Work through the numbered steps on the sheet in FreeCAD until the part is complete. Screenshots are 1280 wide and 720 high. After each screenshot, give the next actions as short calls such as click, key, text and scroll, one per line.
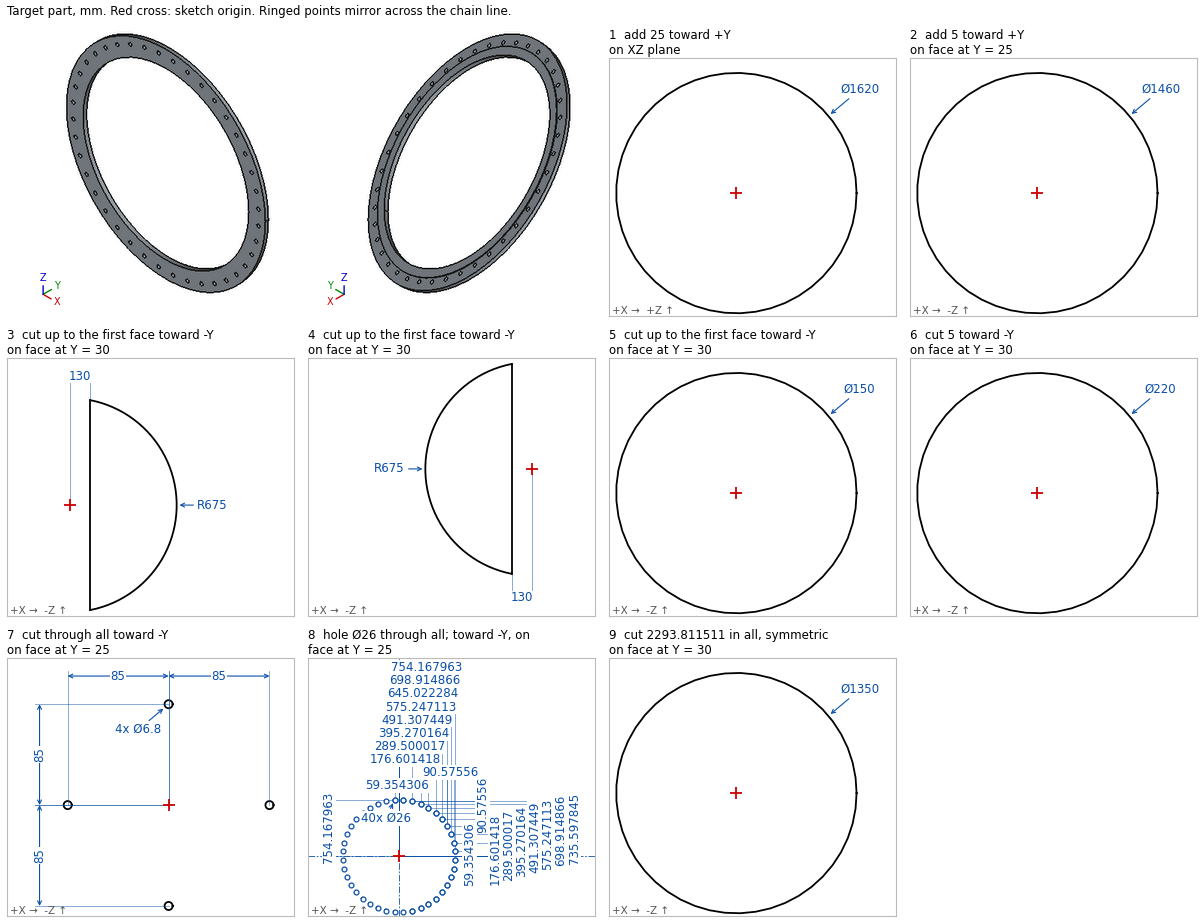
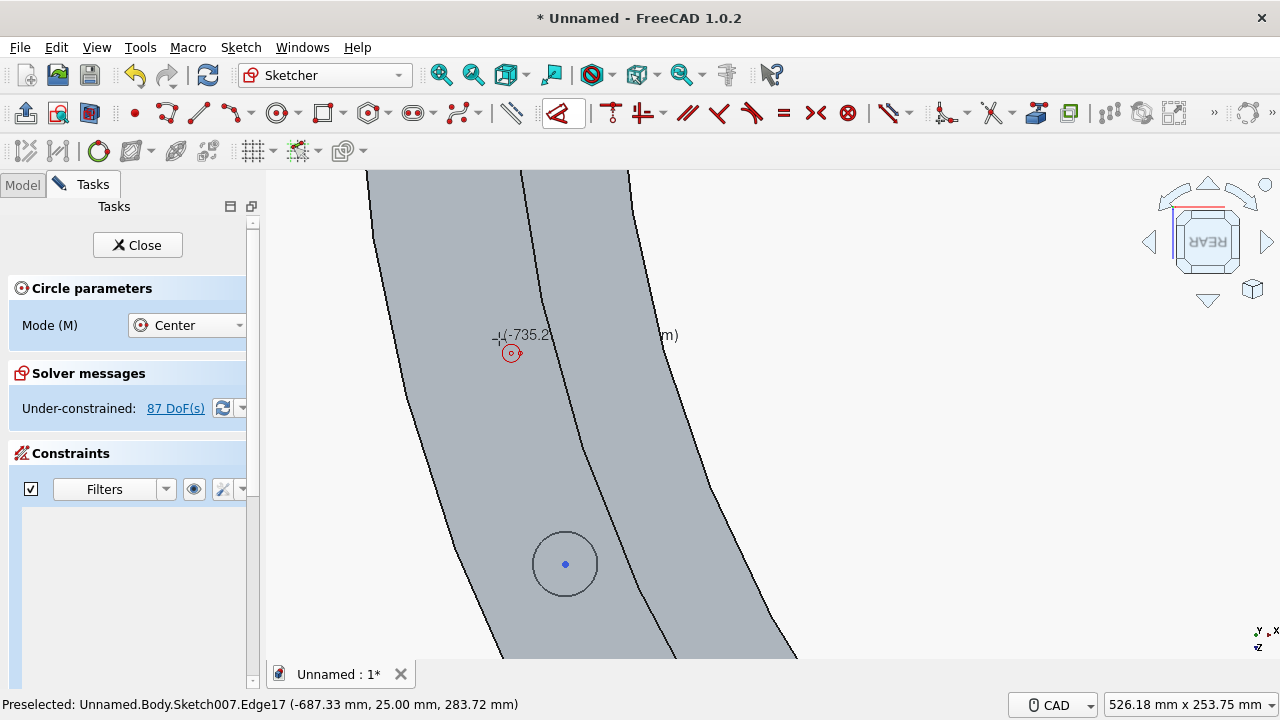
scroll(554, 466, down, 11)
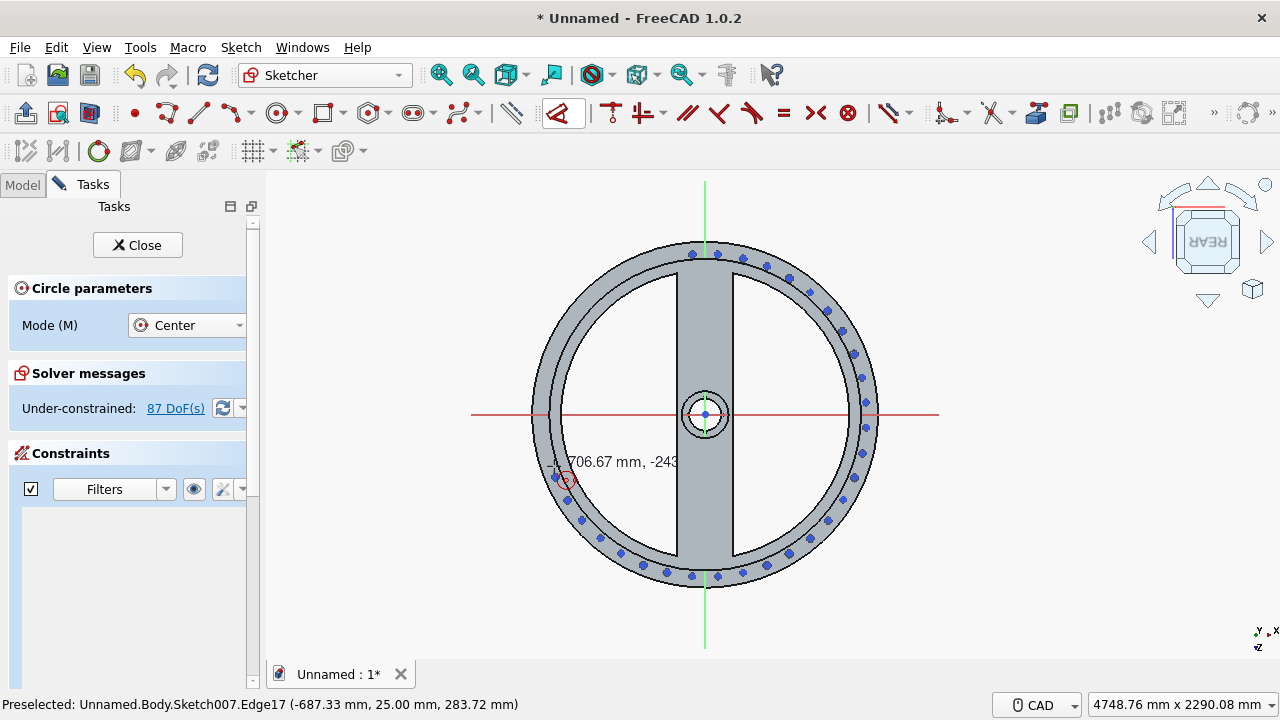
click(548, 452)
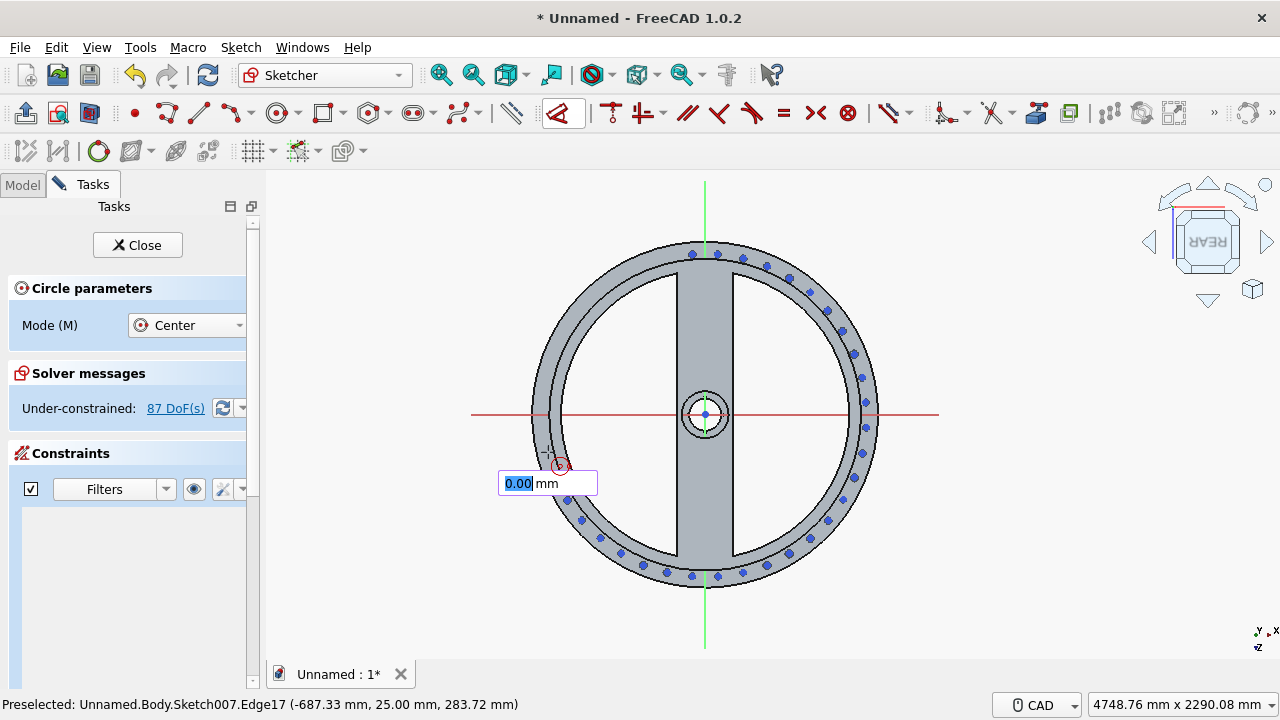
scroll(550, 450, up, 9)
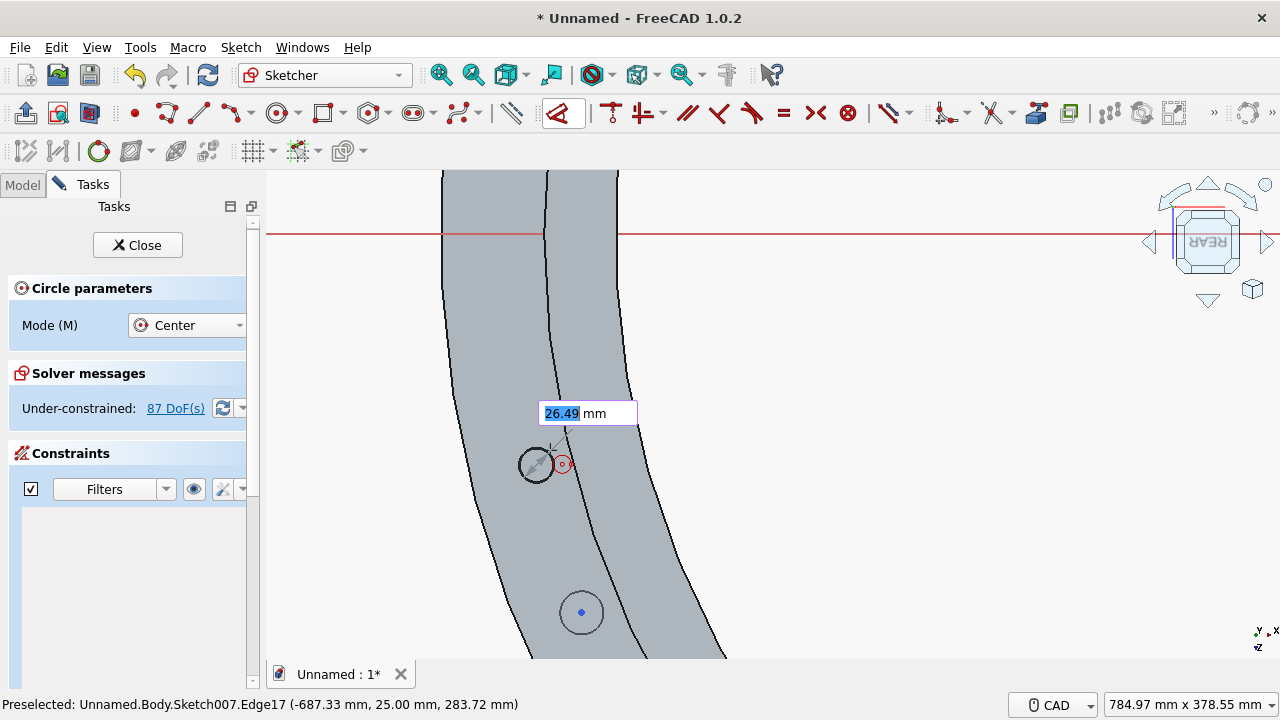
click(549, 450)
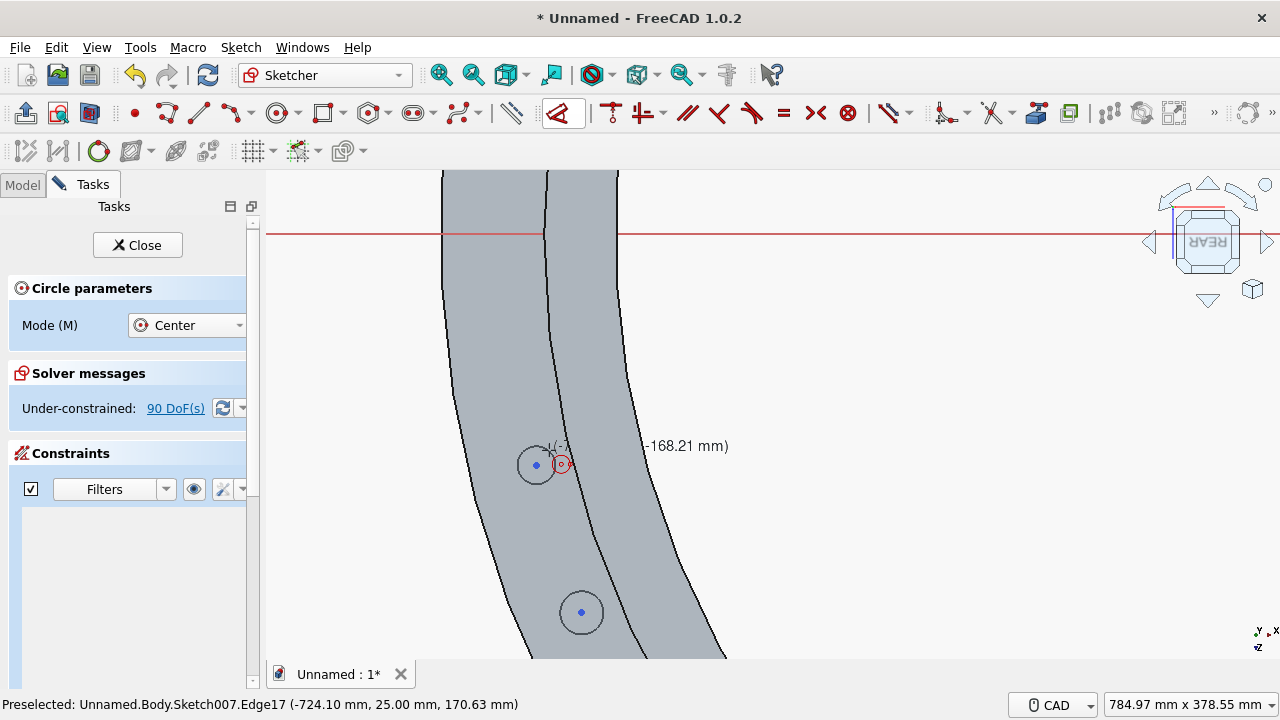
scroll(513, 310, up, 2)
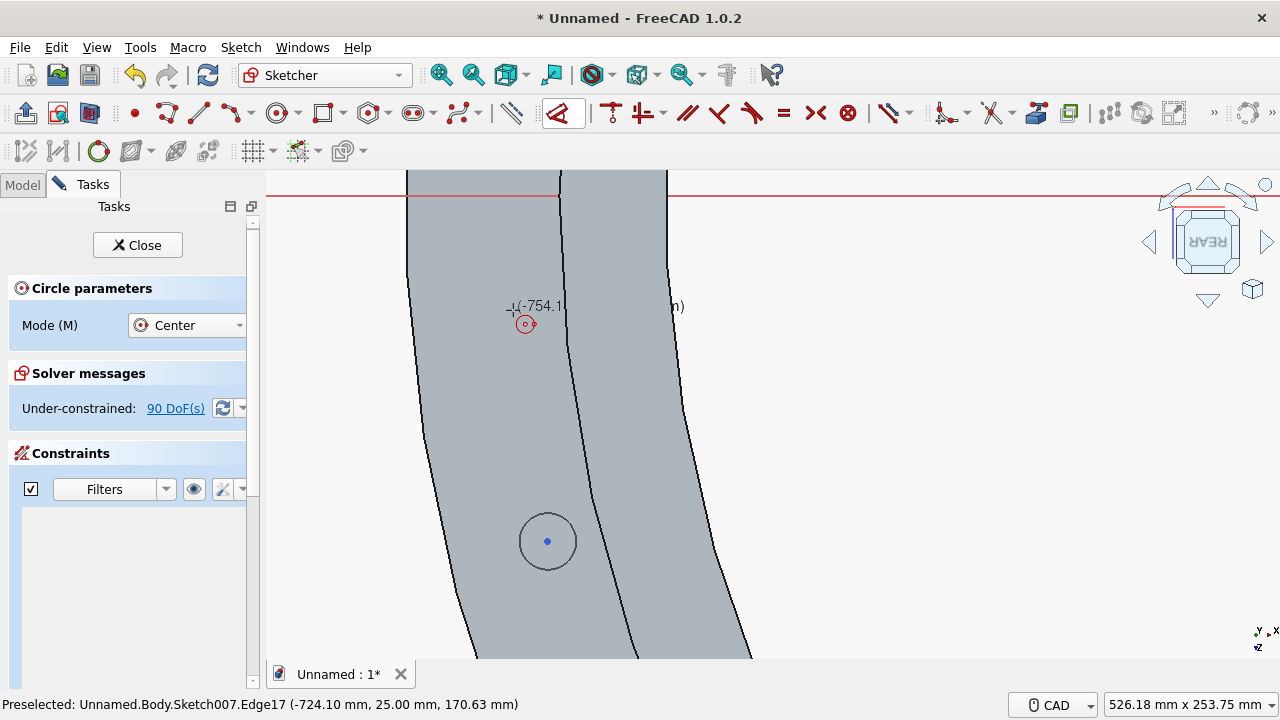
scroll(547, 442, down, 11)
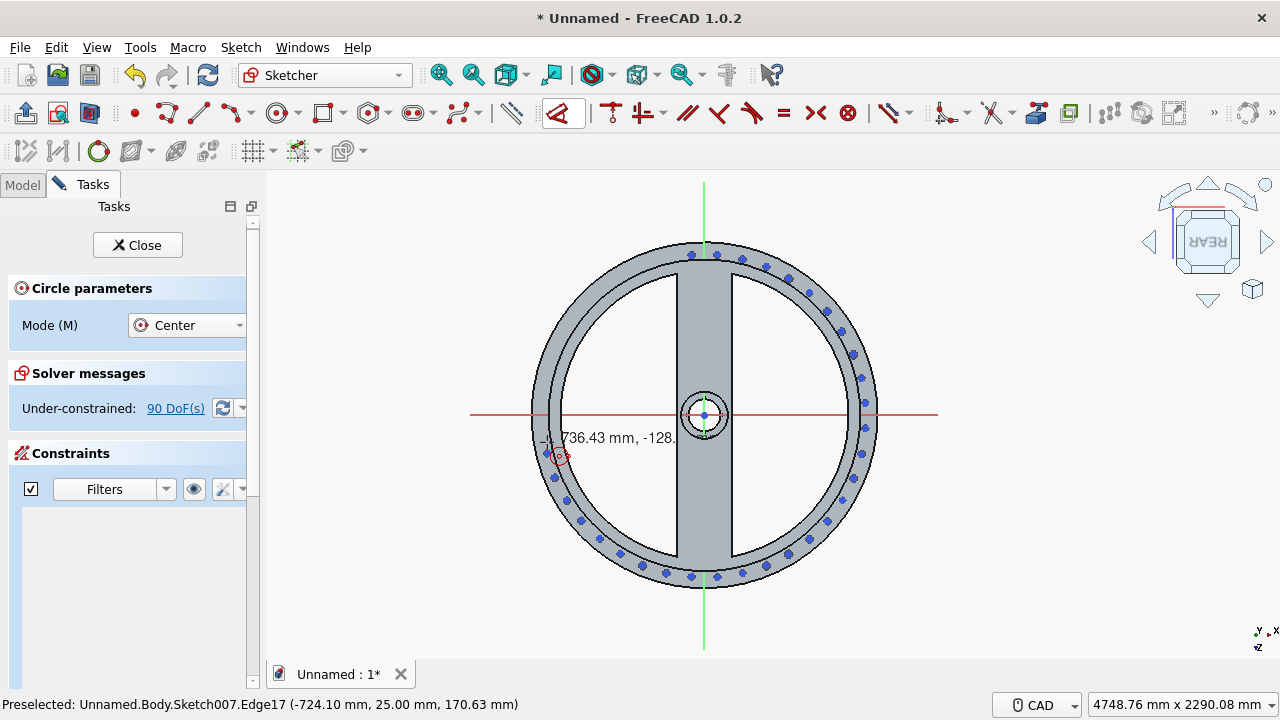
scroll(543, 428, up, 2)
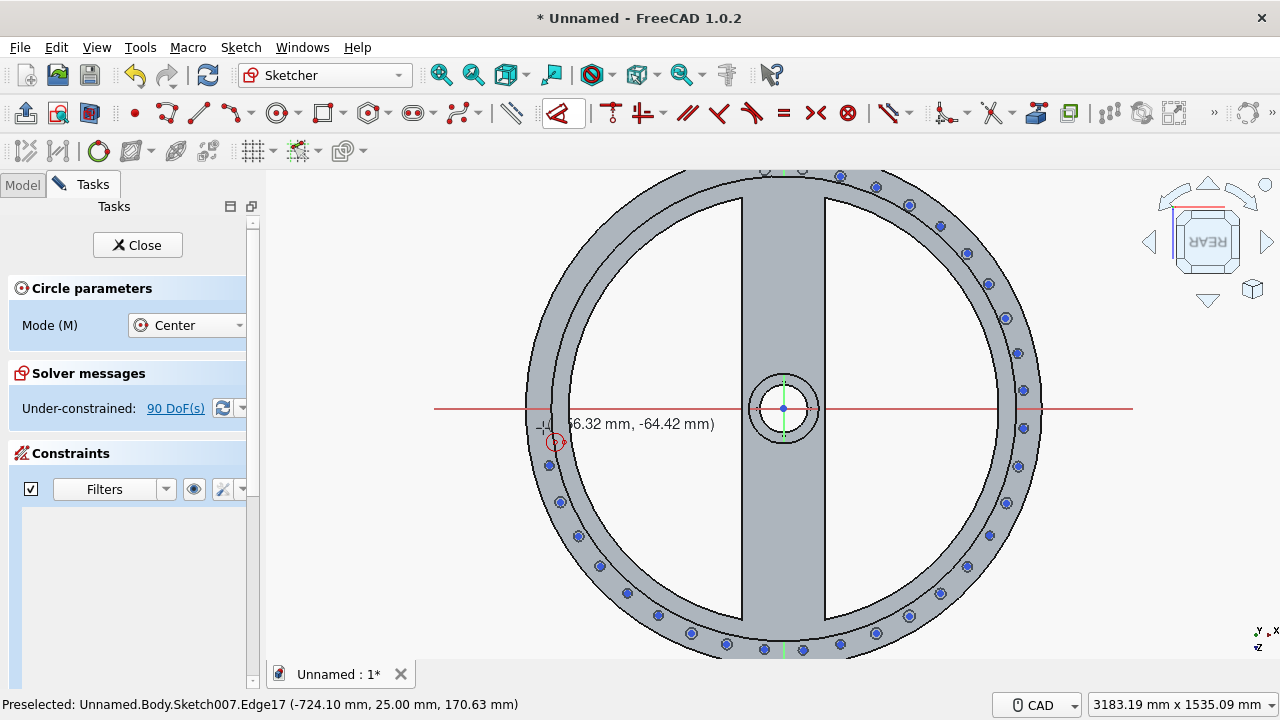
click(544, 428)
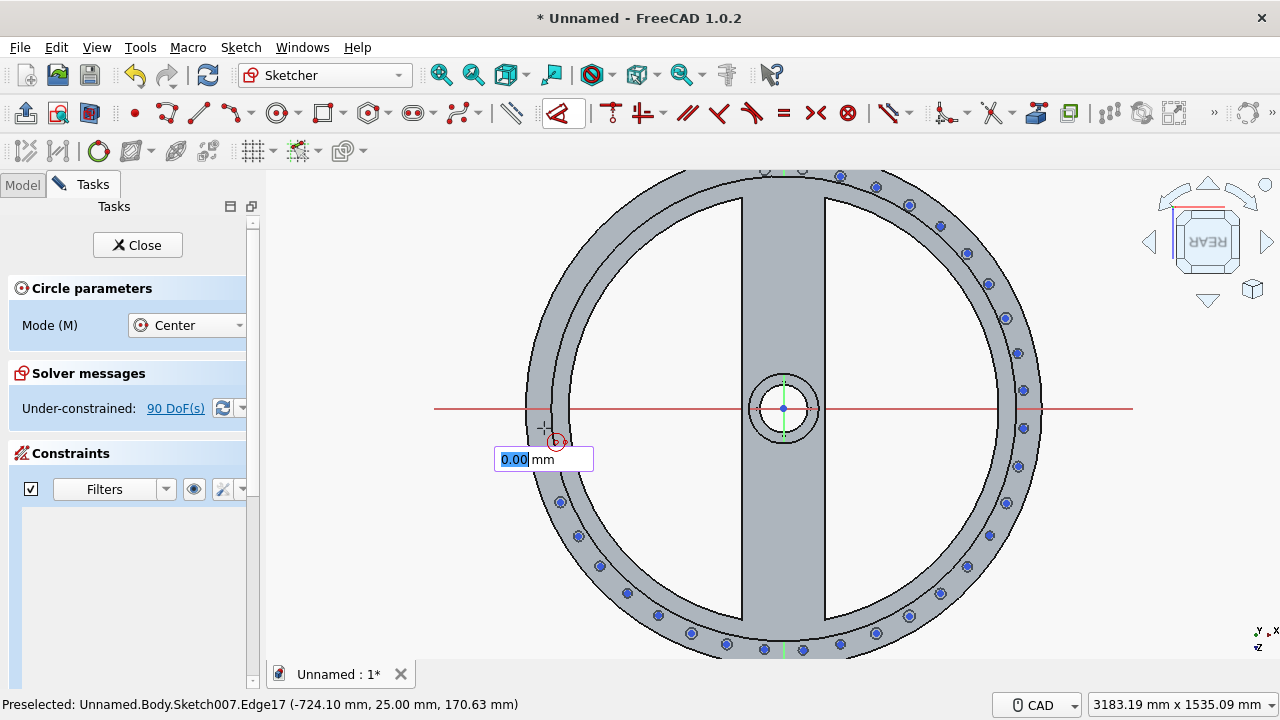
scroll(546, 425, up, 7)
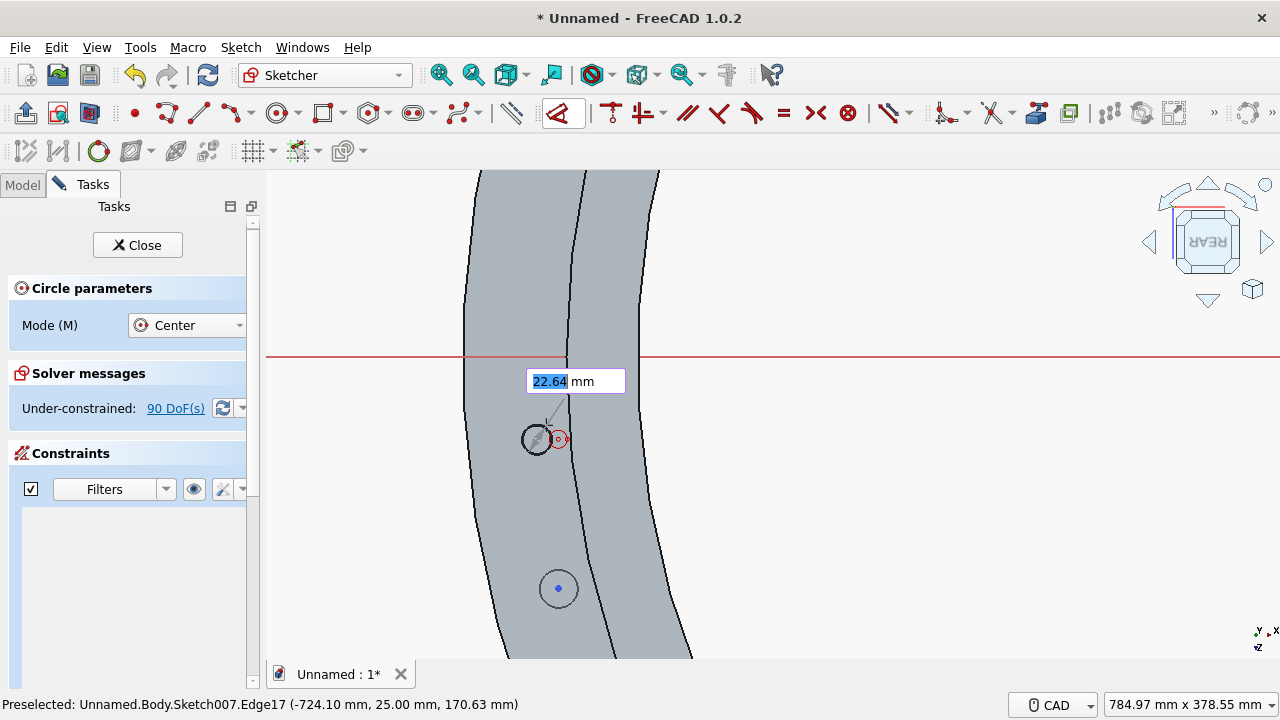
click(547, 422)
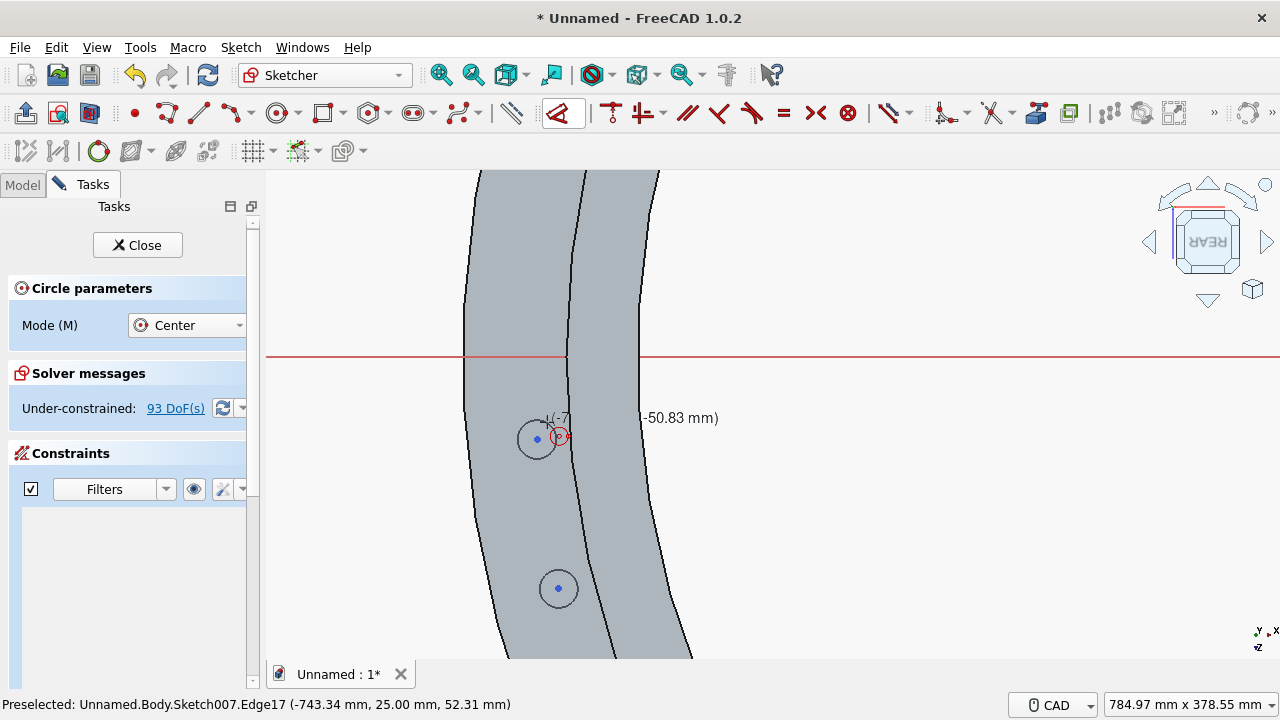
scroll(535, 281, up, 2)